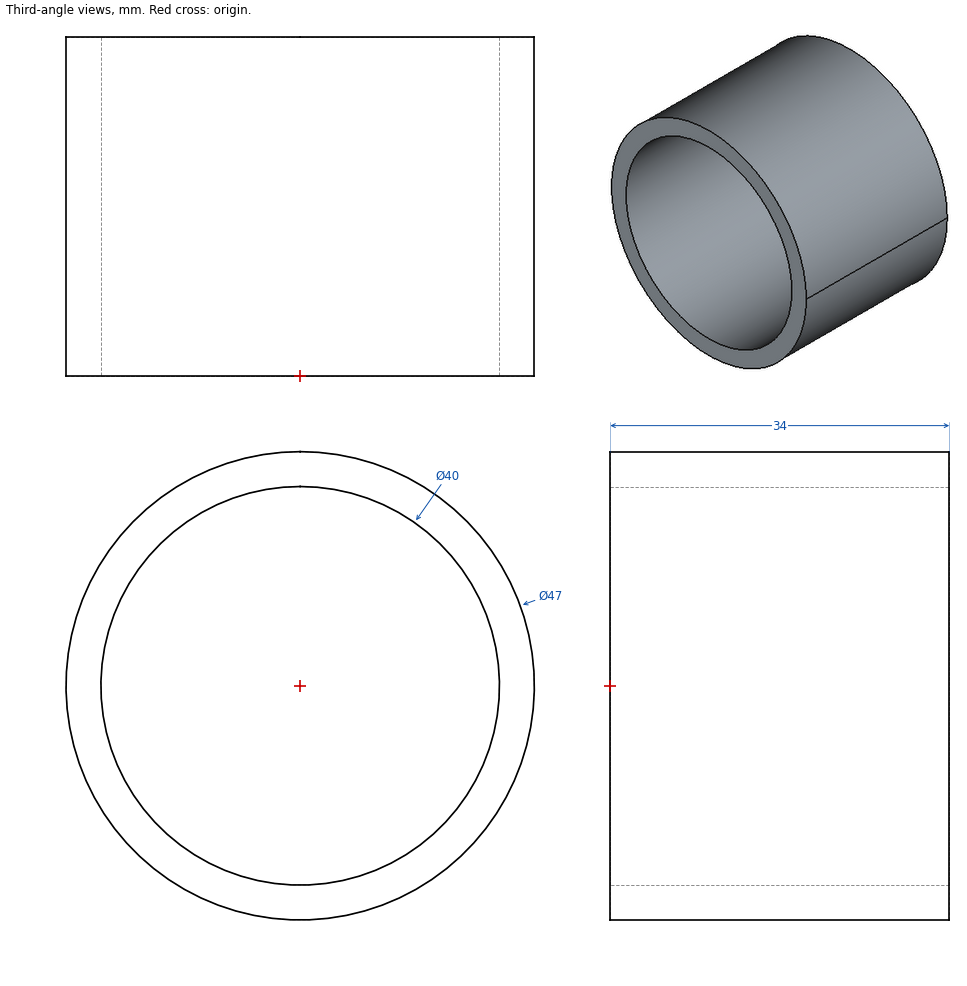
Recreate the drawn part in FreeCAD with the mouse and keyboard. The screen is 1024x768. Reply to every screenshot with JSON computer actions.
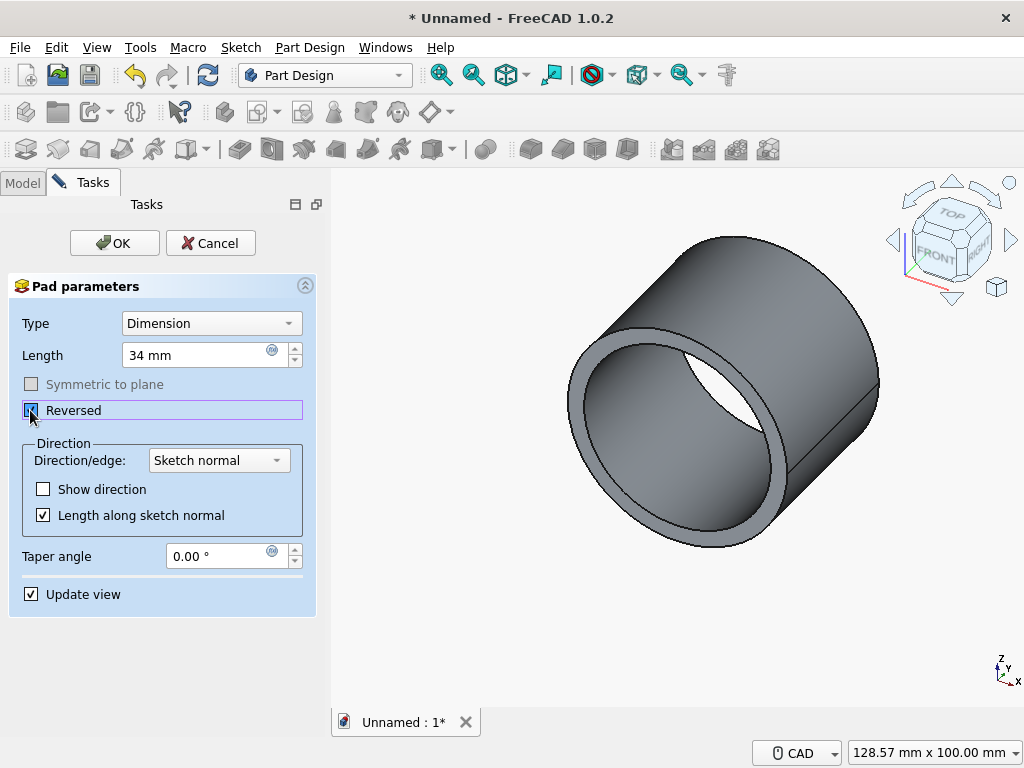
{"action": "left_click", "coordinate": [115, 243]}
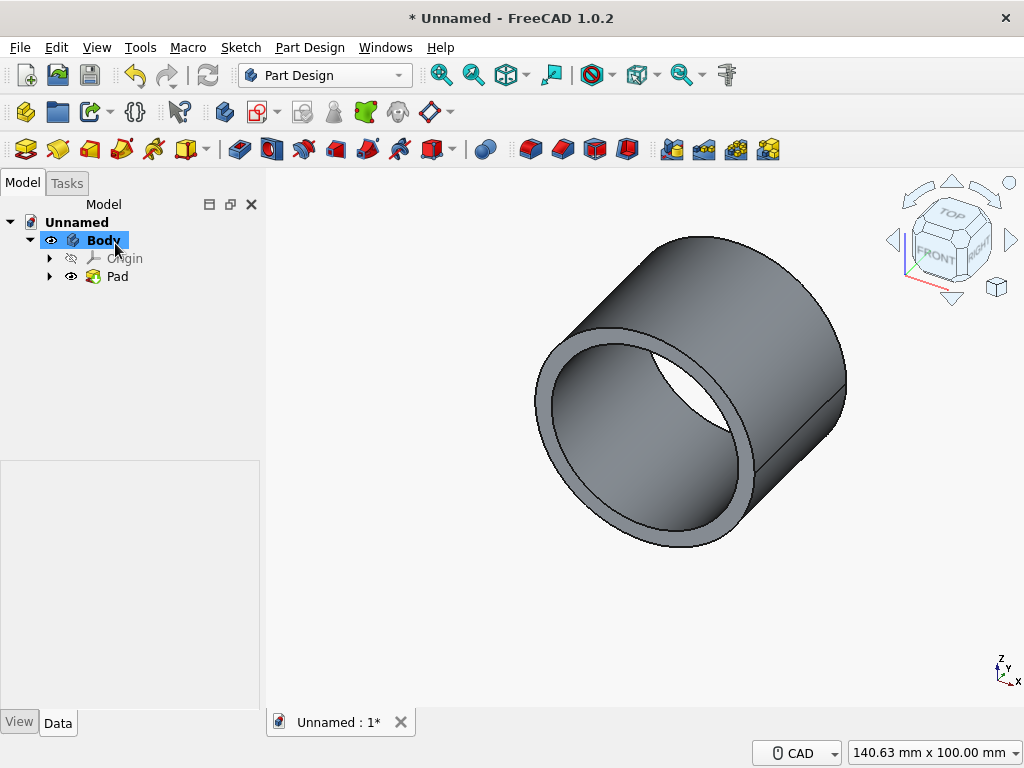
{"action": "key", "text": "0"}